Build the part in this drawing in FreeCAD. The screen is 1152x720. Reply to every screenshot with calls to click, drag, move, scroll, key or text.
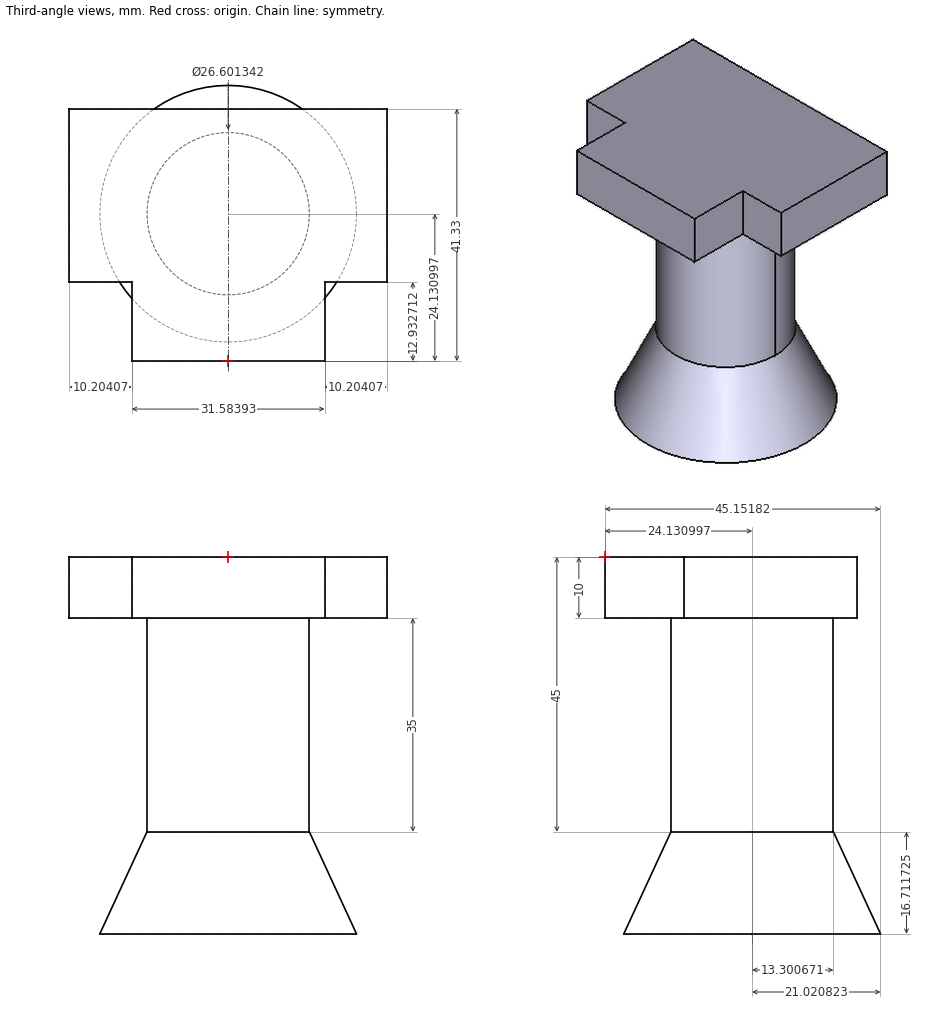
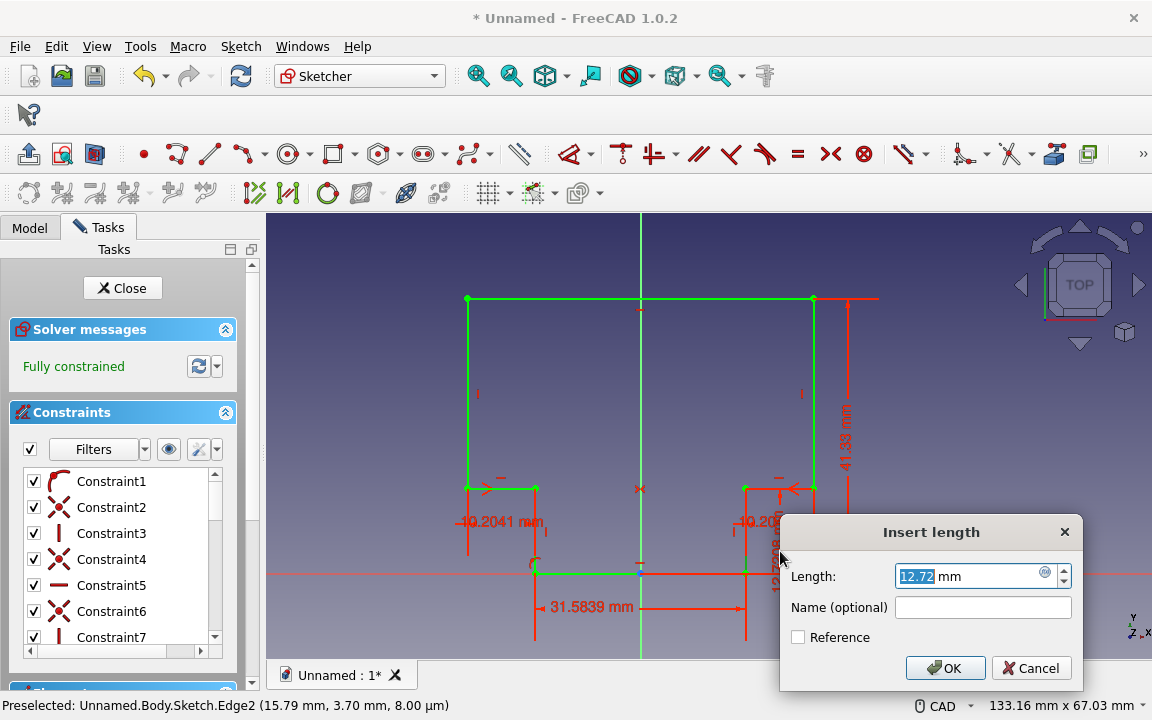
text(12.932712)
key(Return)
key(Escape)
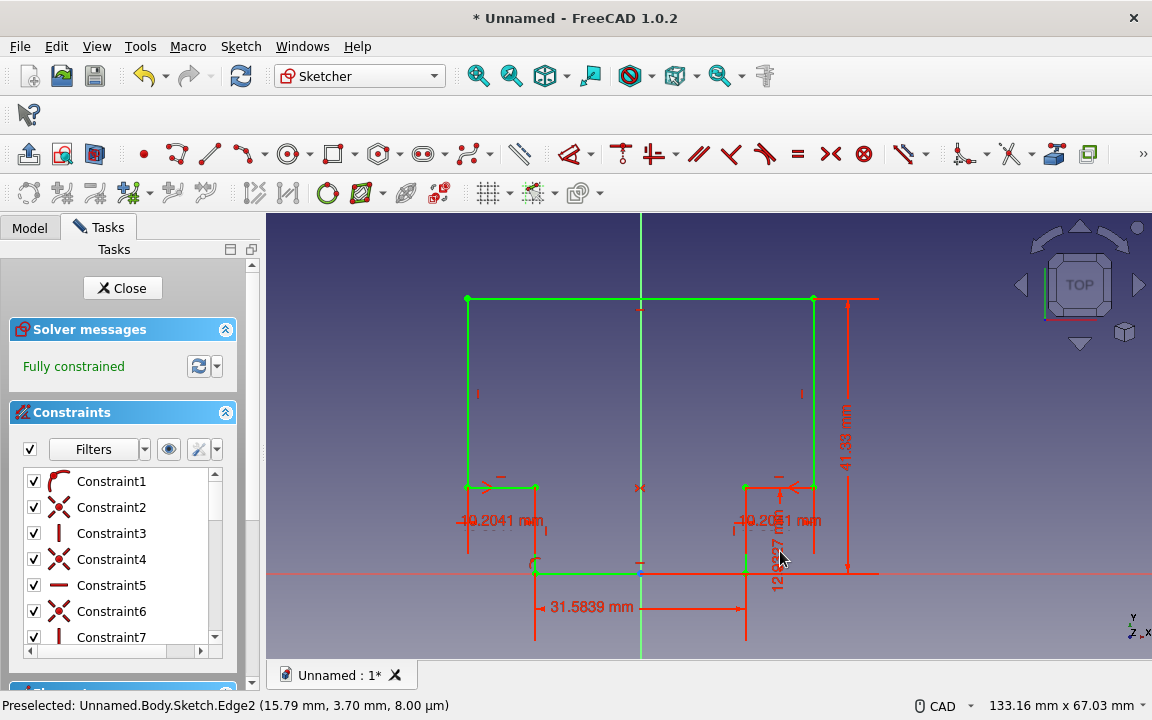
click(123, 288)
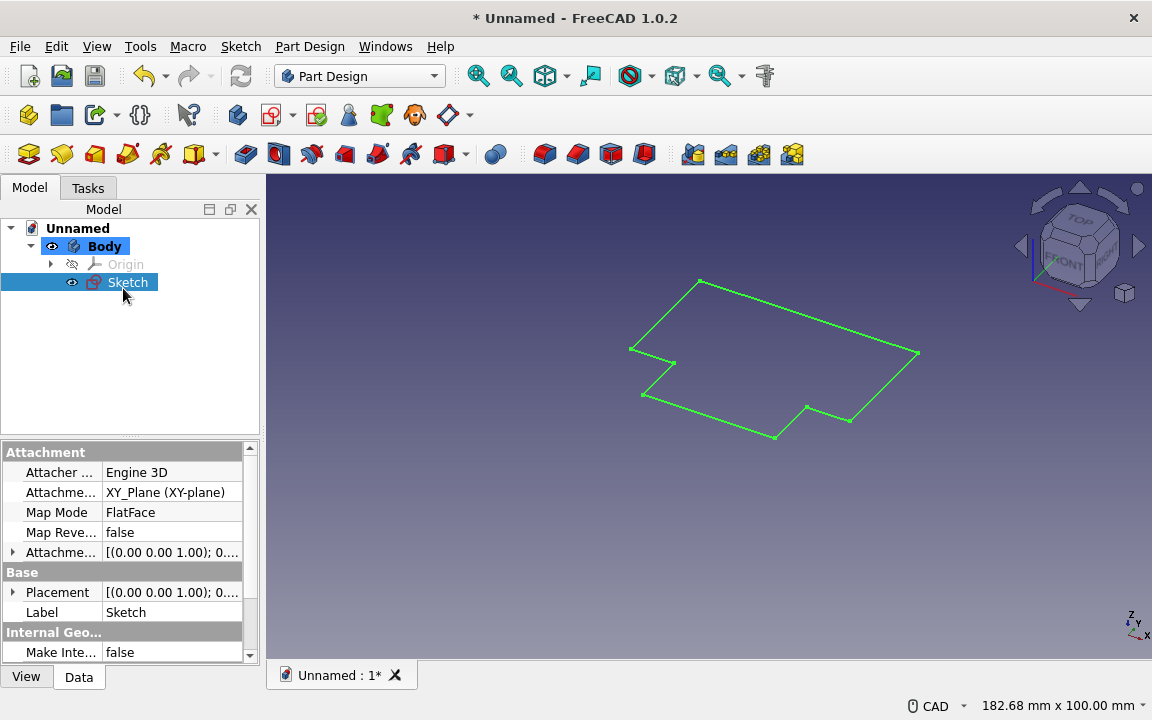
click(29, 154)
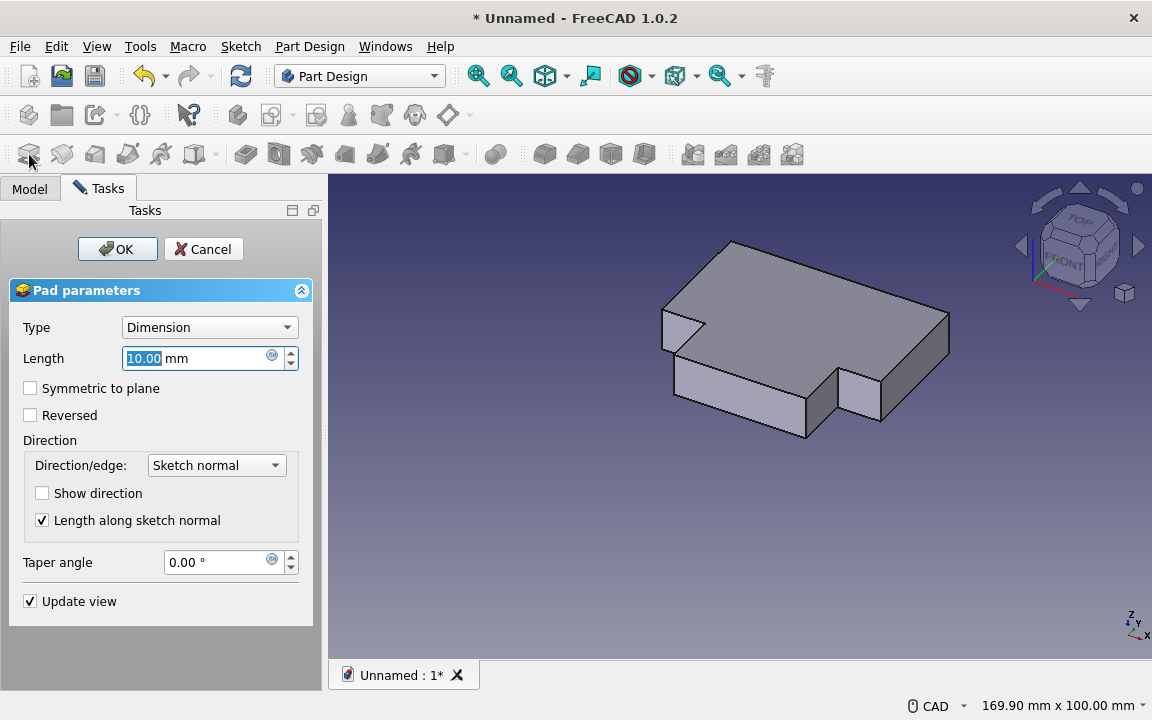
text(10)
key(Tab)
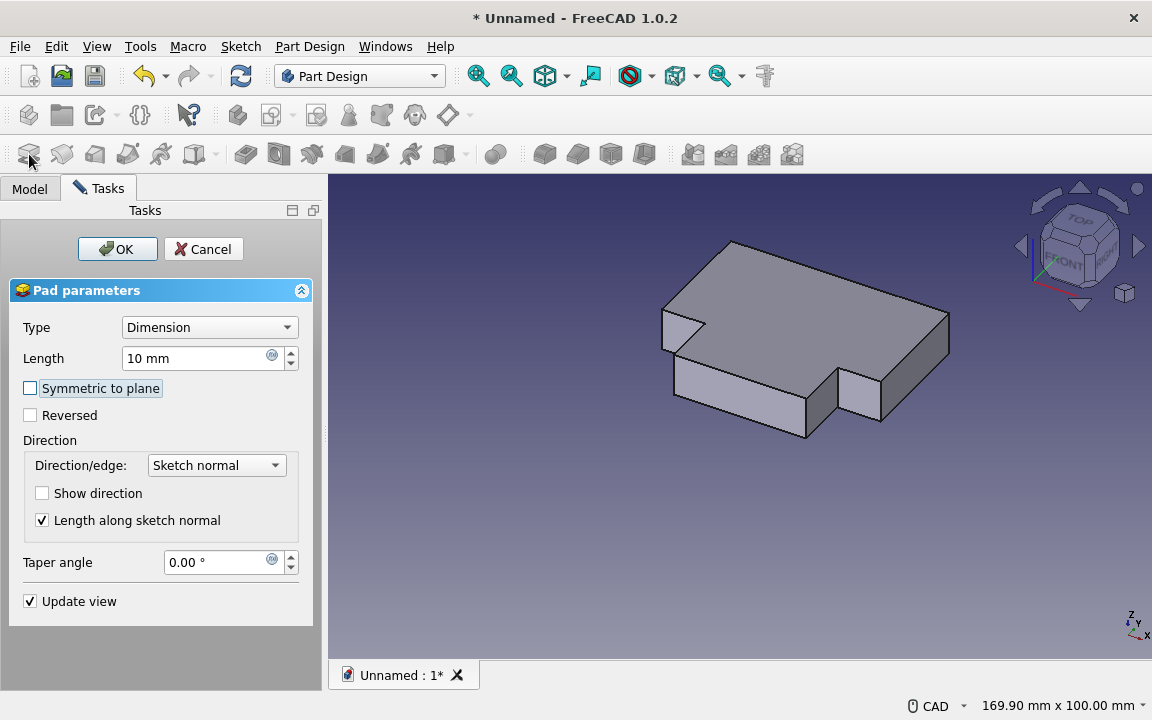
click(31, 415)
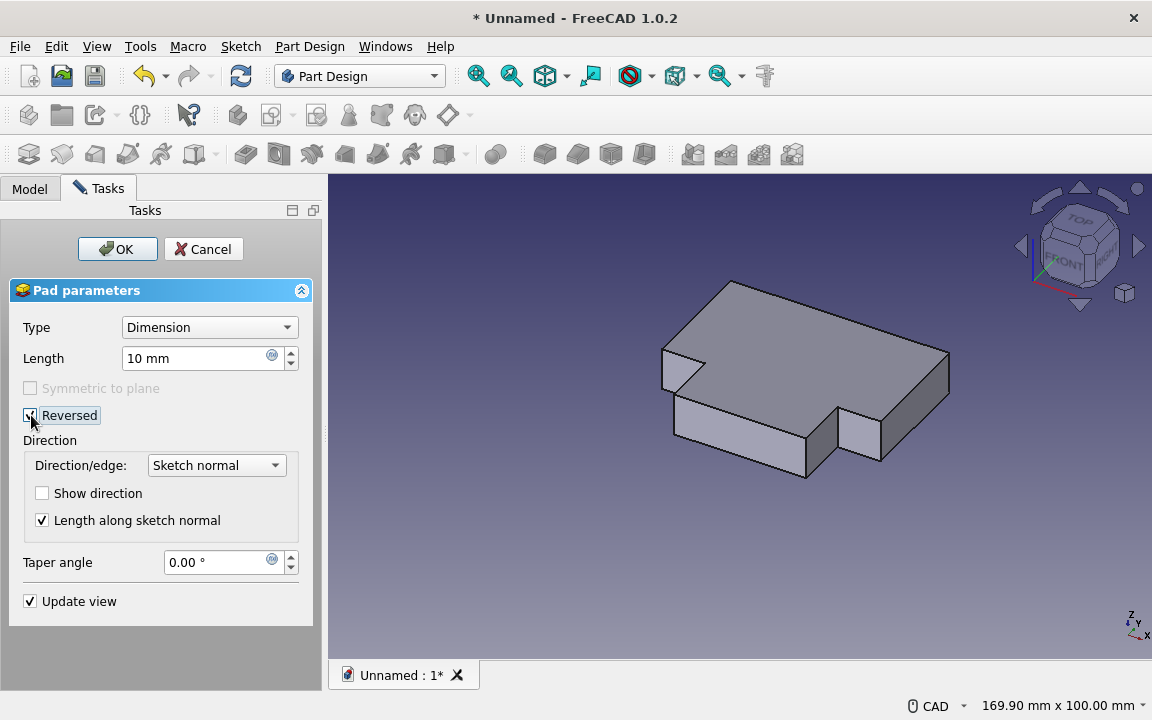
click(118, 249)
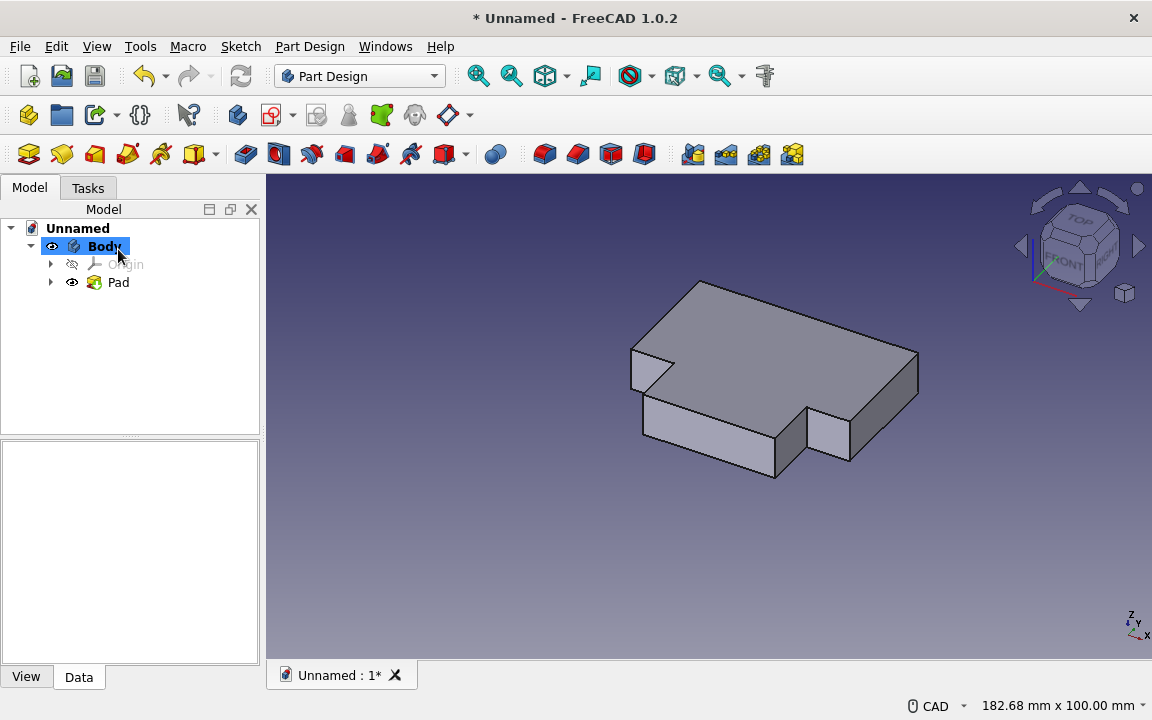
click(479, 76)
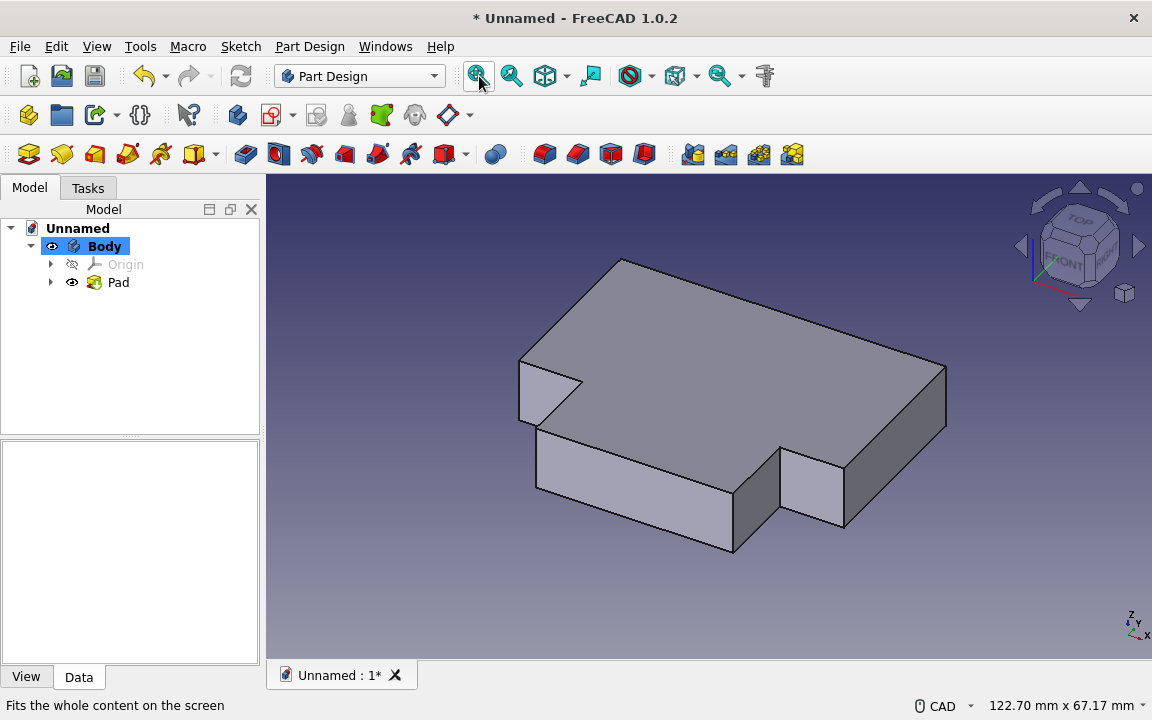
key(5)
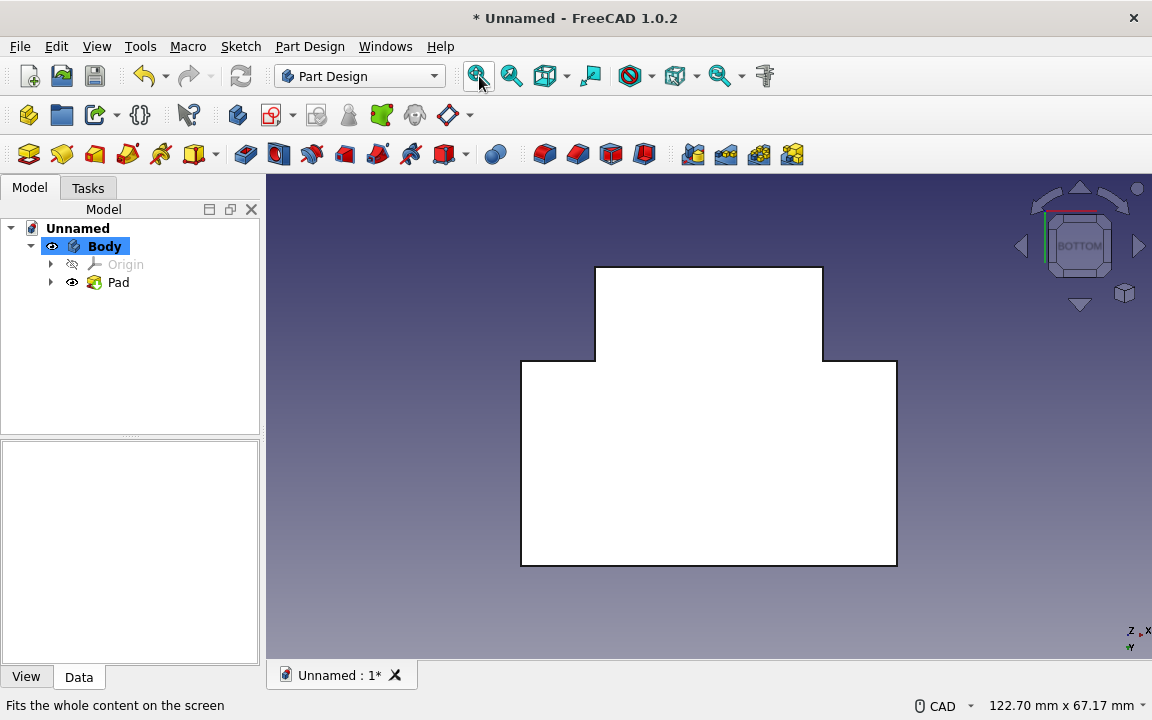
click(709, 415)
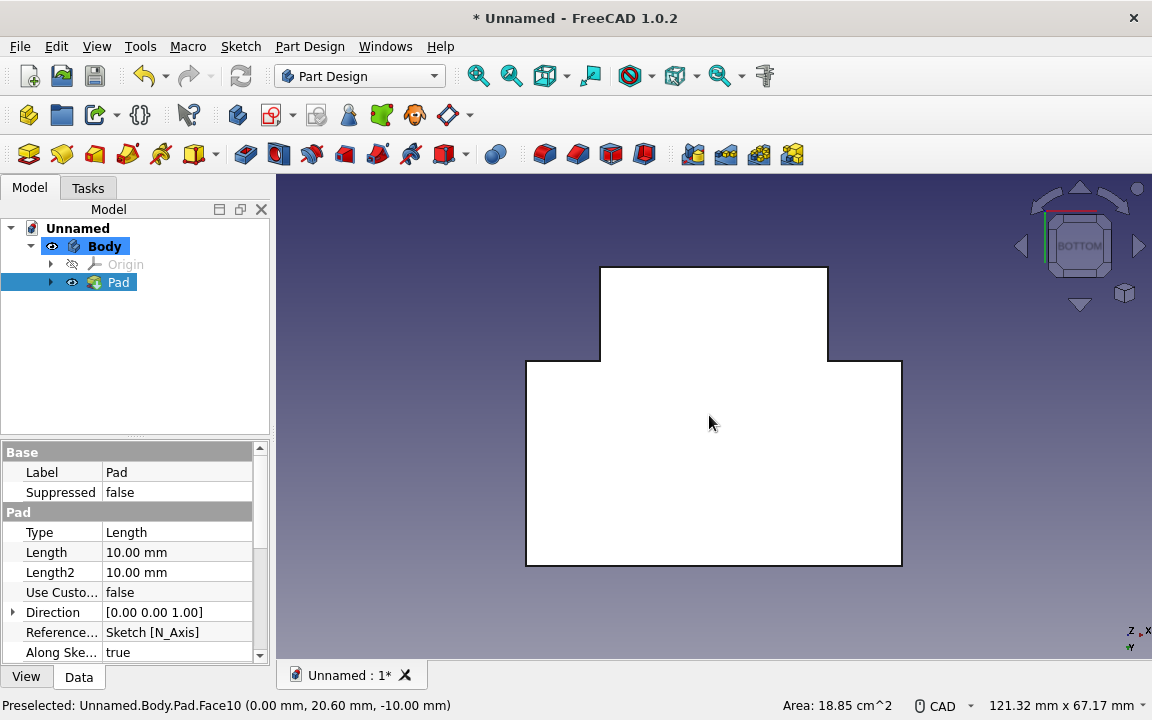
click(270, 116)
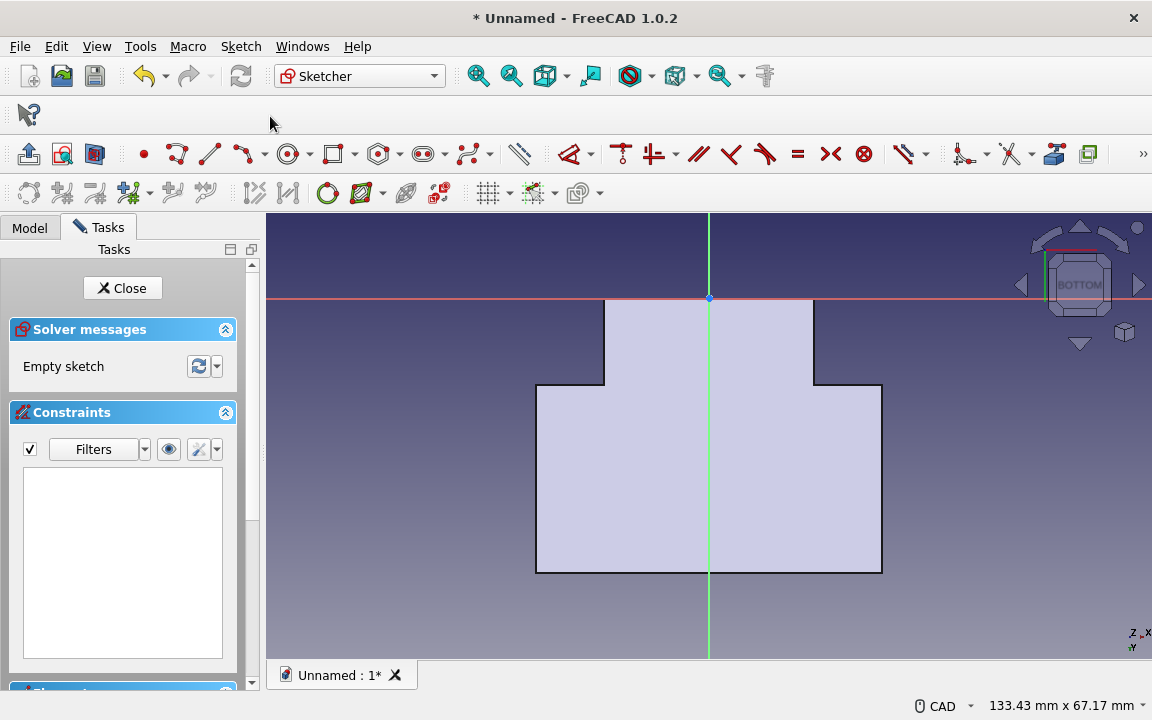
click(288, 154)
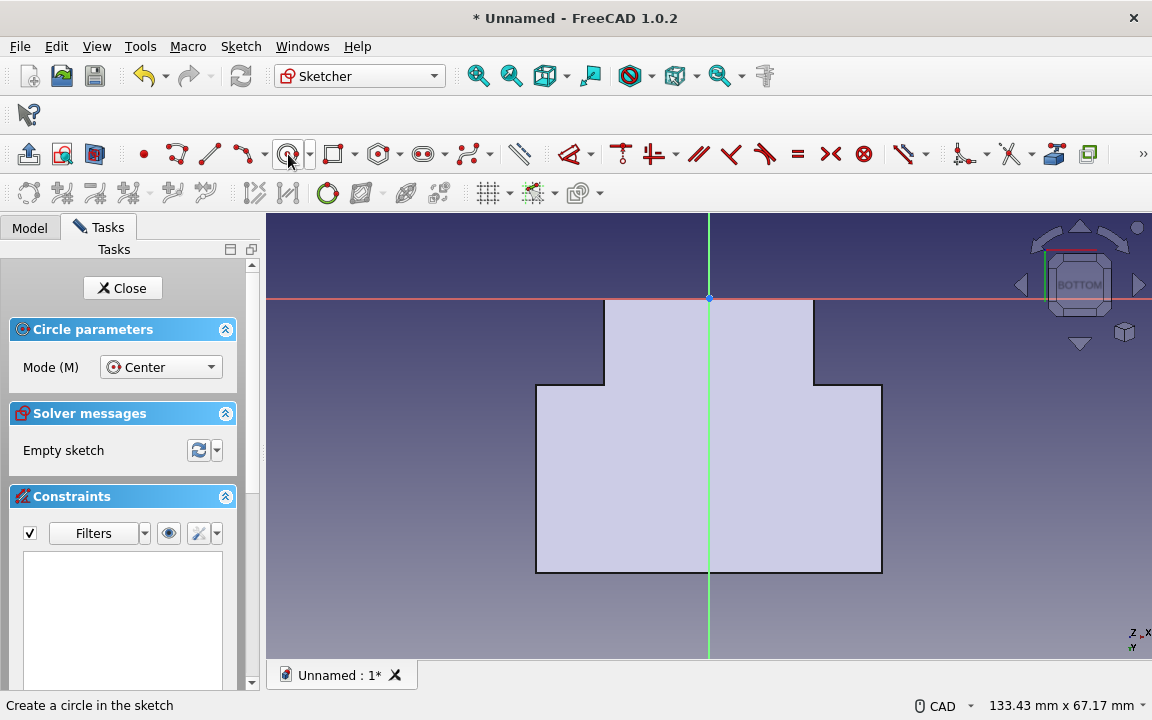
click(709, 459)
click(771, 397)
key(Escape)